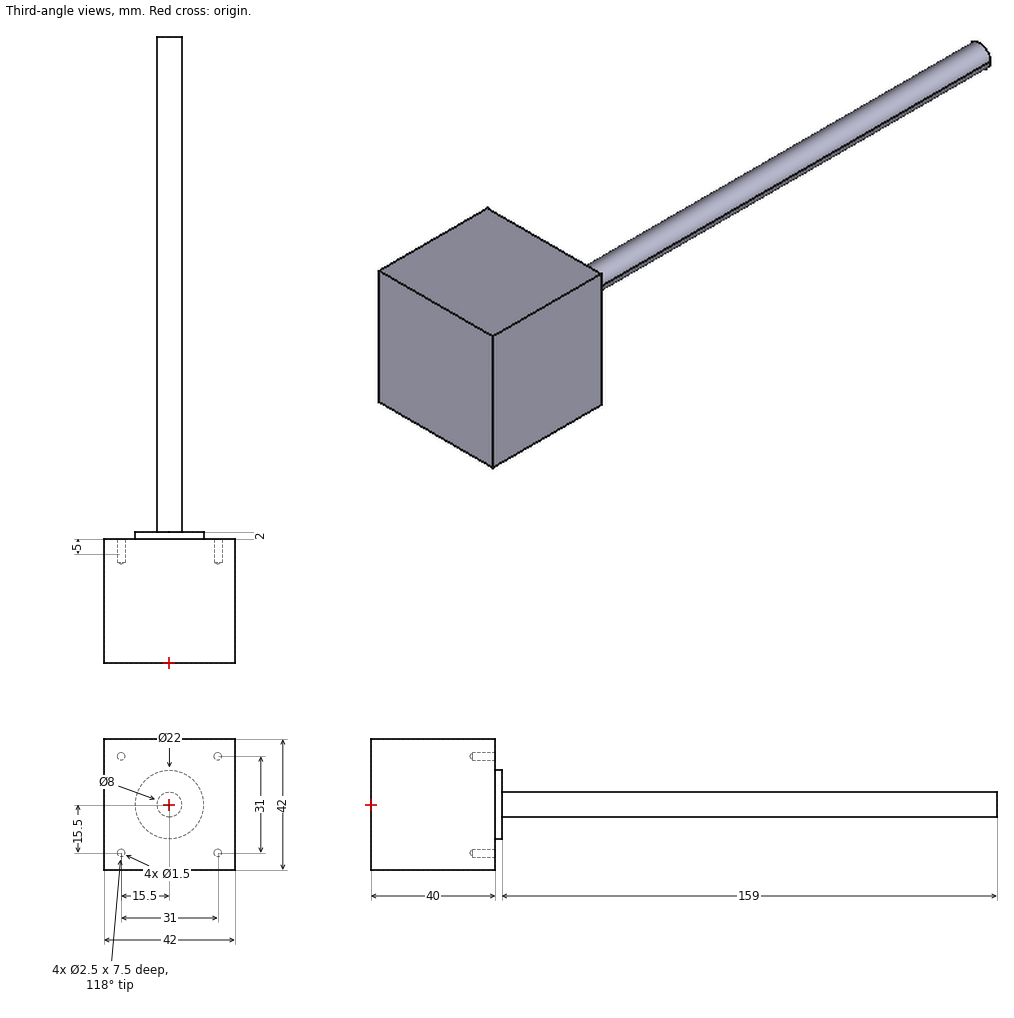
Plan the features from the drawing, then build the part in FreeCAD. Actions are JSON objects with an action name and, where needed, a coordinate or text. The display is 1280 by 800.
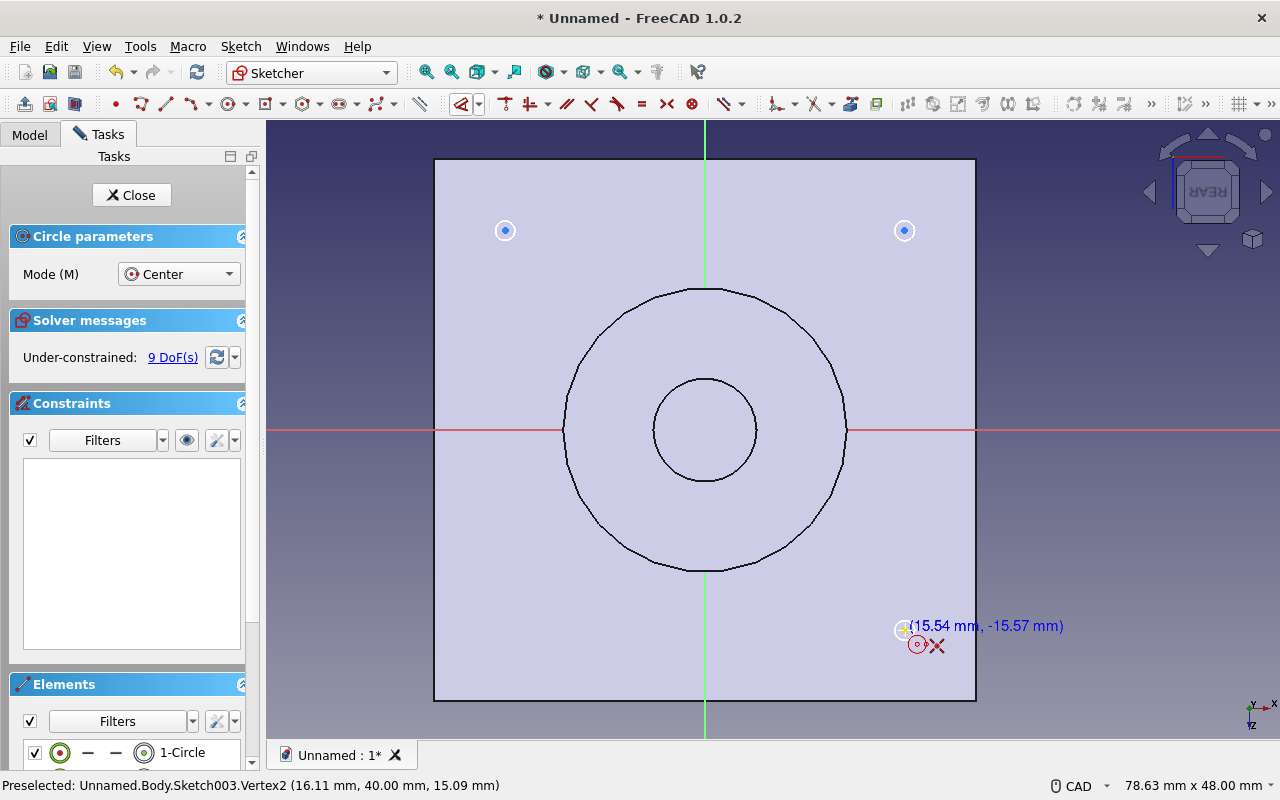
{"action": "scroll", "coordinate": [505, 630], "scroll_direction": "up", "scroll_amount": 5}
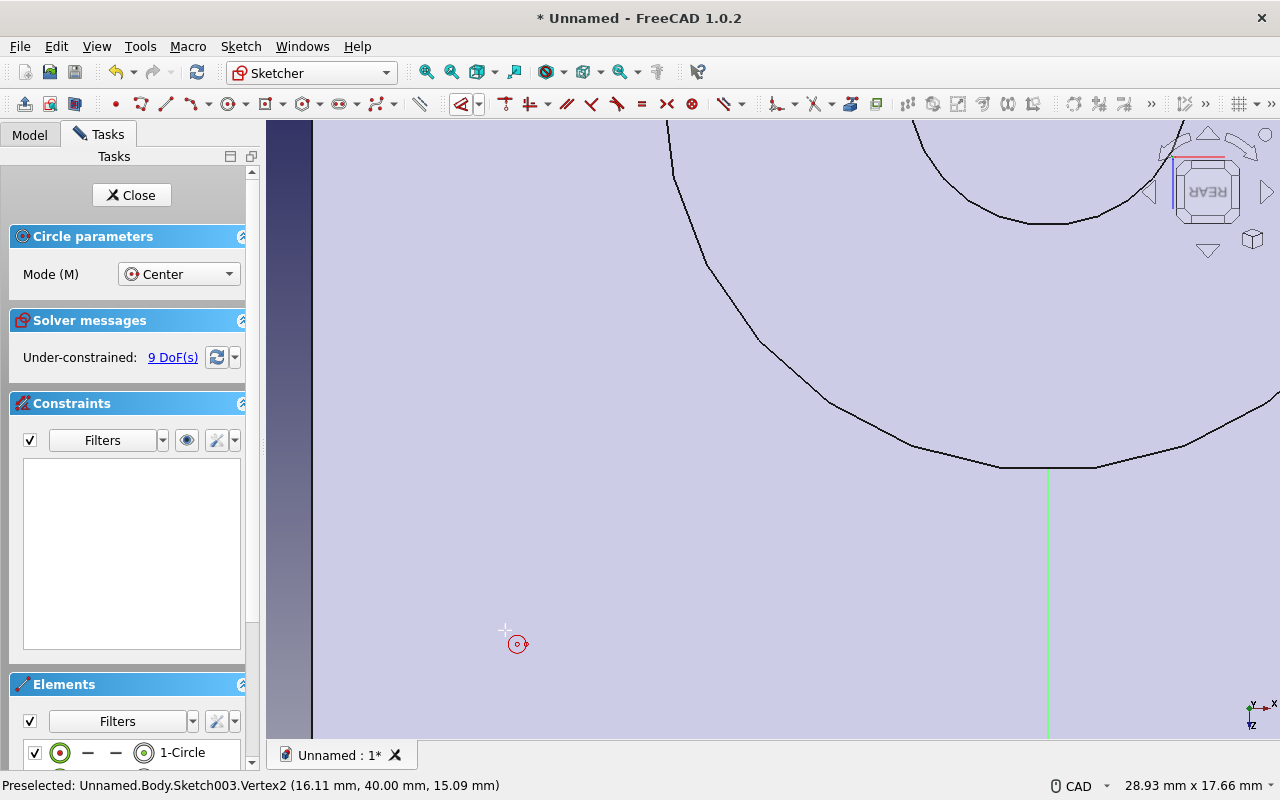
{"action": "left_click", "coordinate": [505, 629]}
{"action": "left_click", "coordinate": [523, 610]}
{"action": "key", "text": "Escape"}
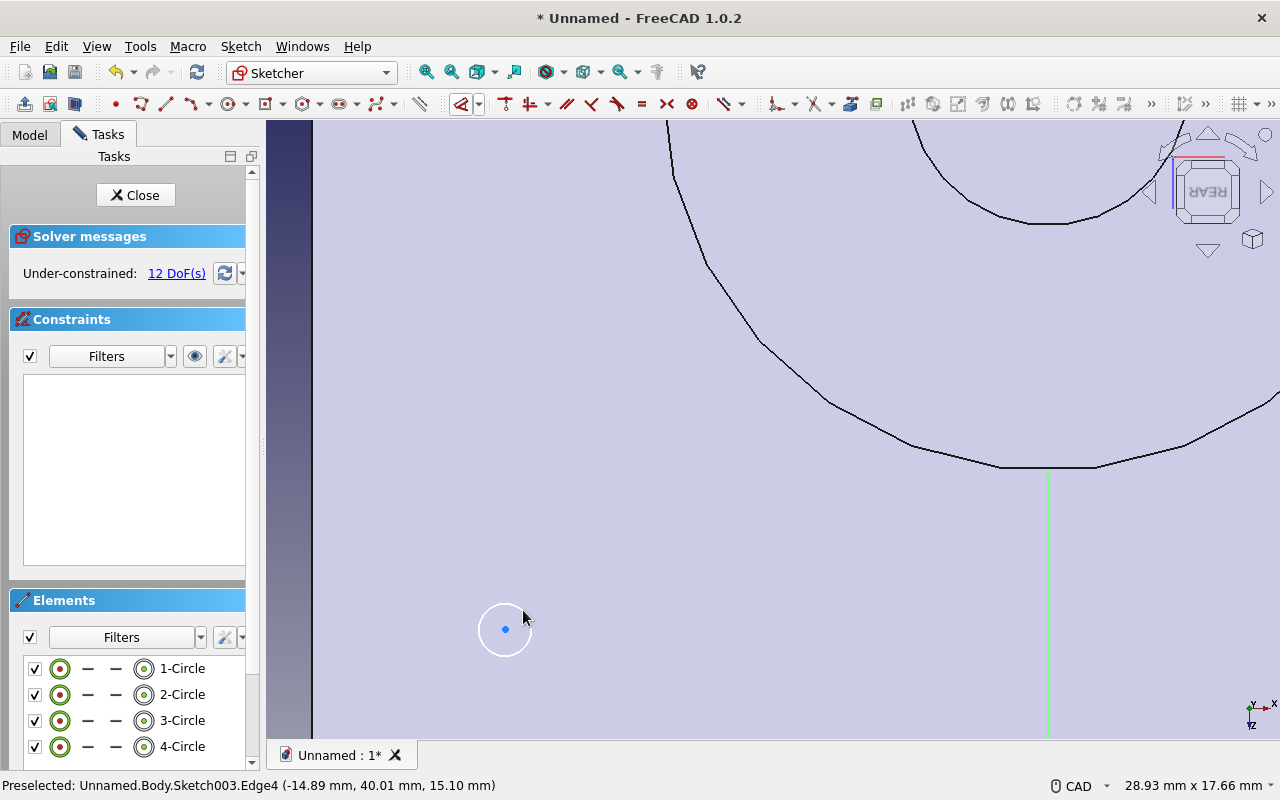
{"action": "scroll", "coordinate": [505, 630], "scroll_direction": "down", "scroll_amount": 5}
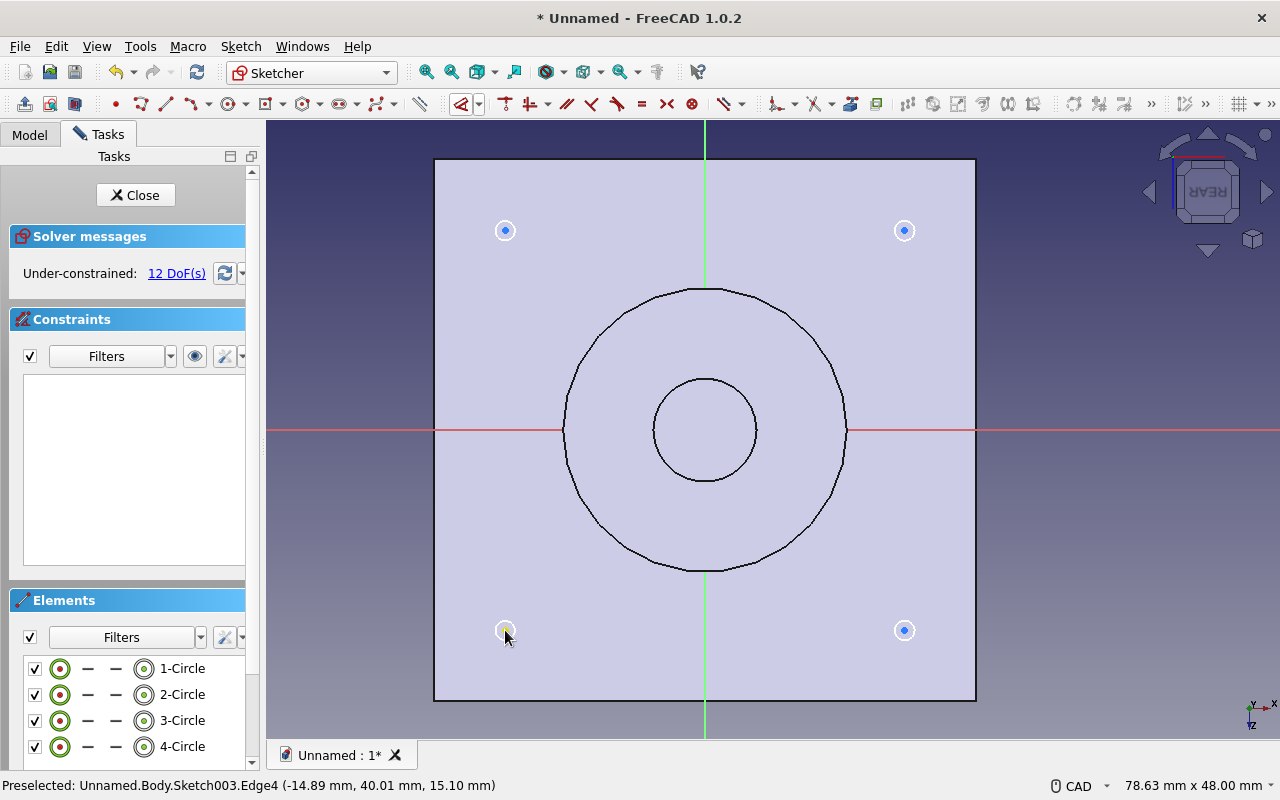
{"action": "scroll", "coordinate": [512, 224], "scroll_direction": "up", "scroll_amount": 2}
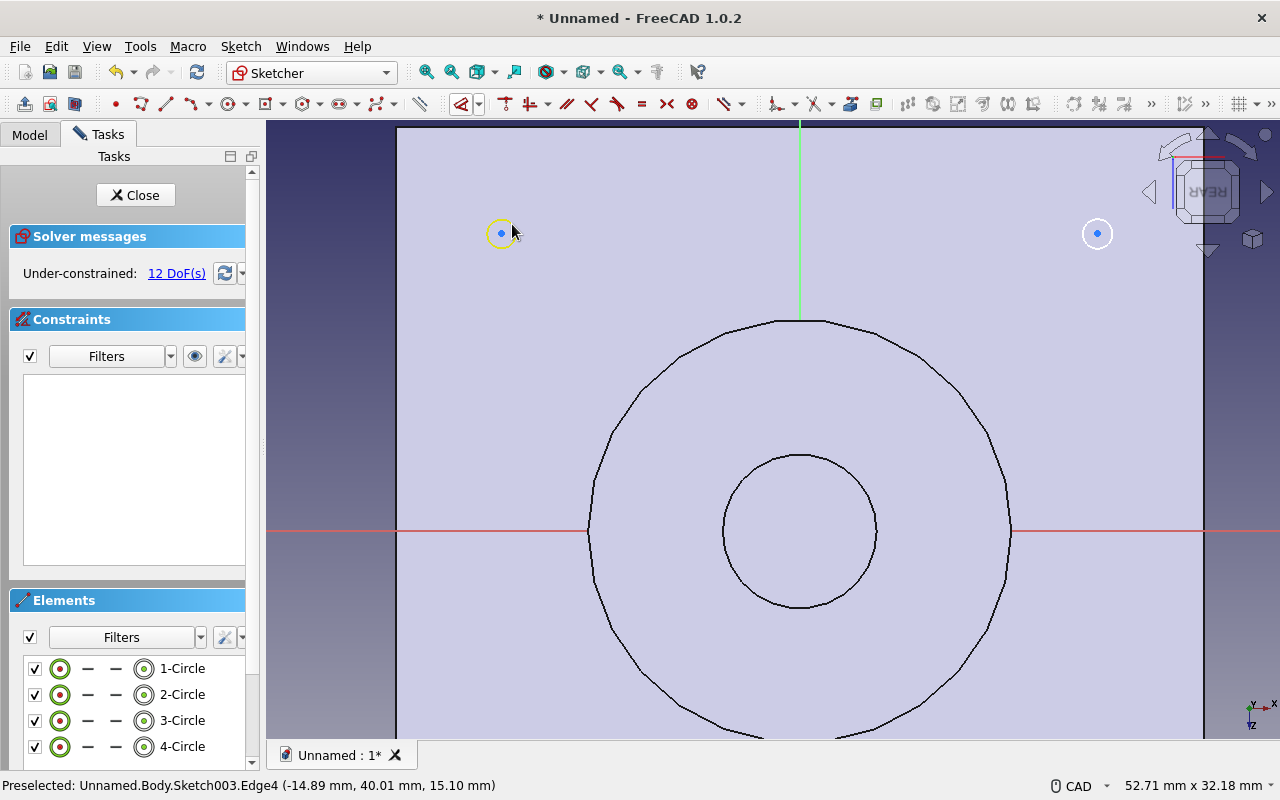
{"action": "left_click", "coordinate": [512, 224]}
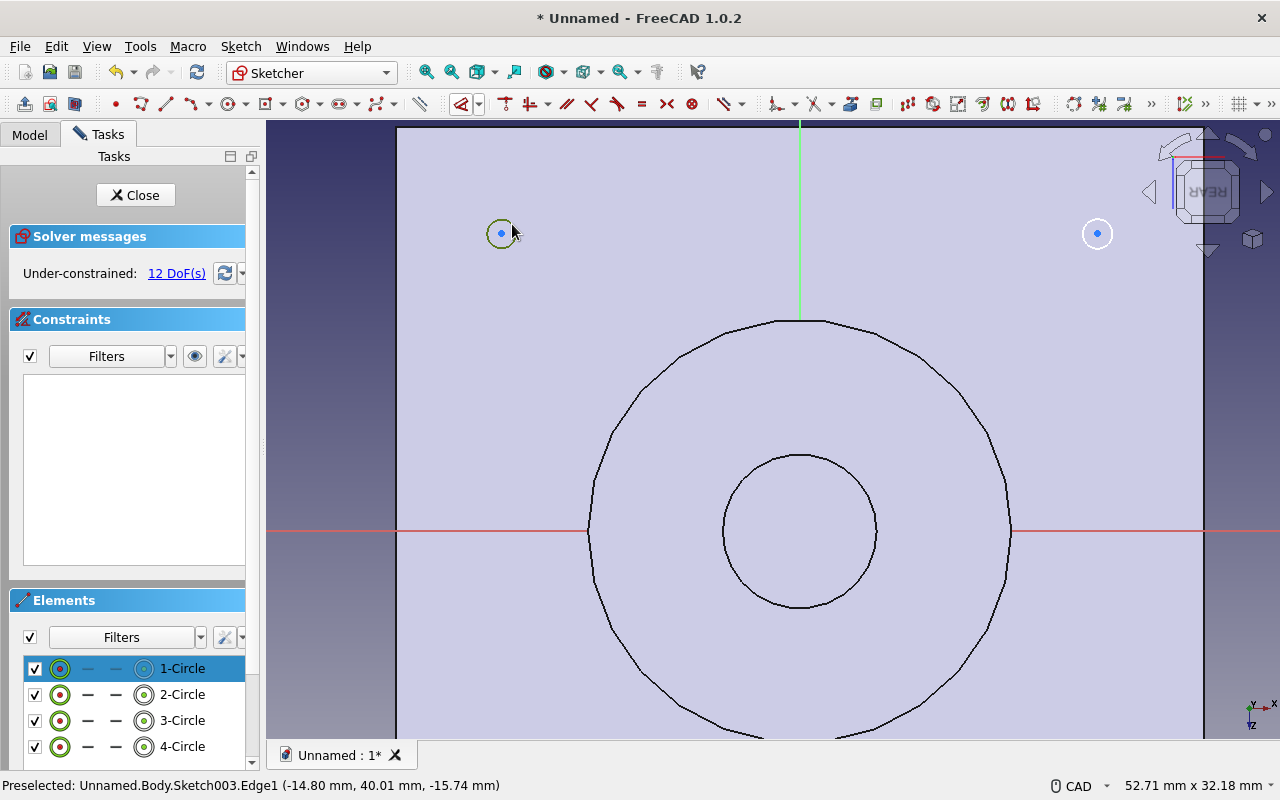
{"action": "left_click", "coordinate": [1108, 224]}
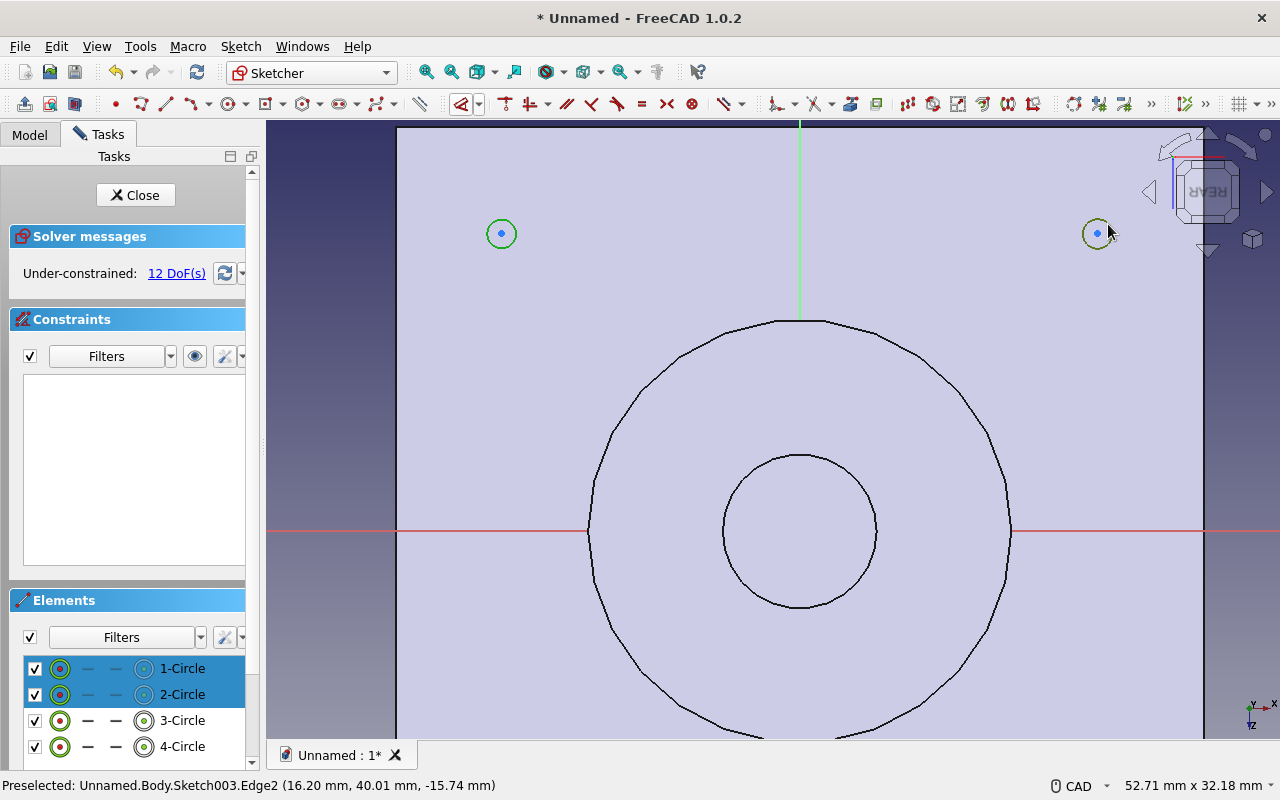
{"action": "scroll", "coordinate": [511, 222], "scroll_direction": "down", "scroll_amount": 2}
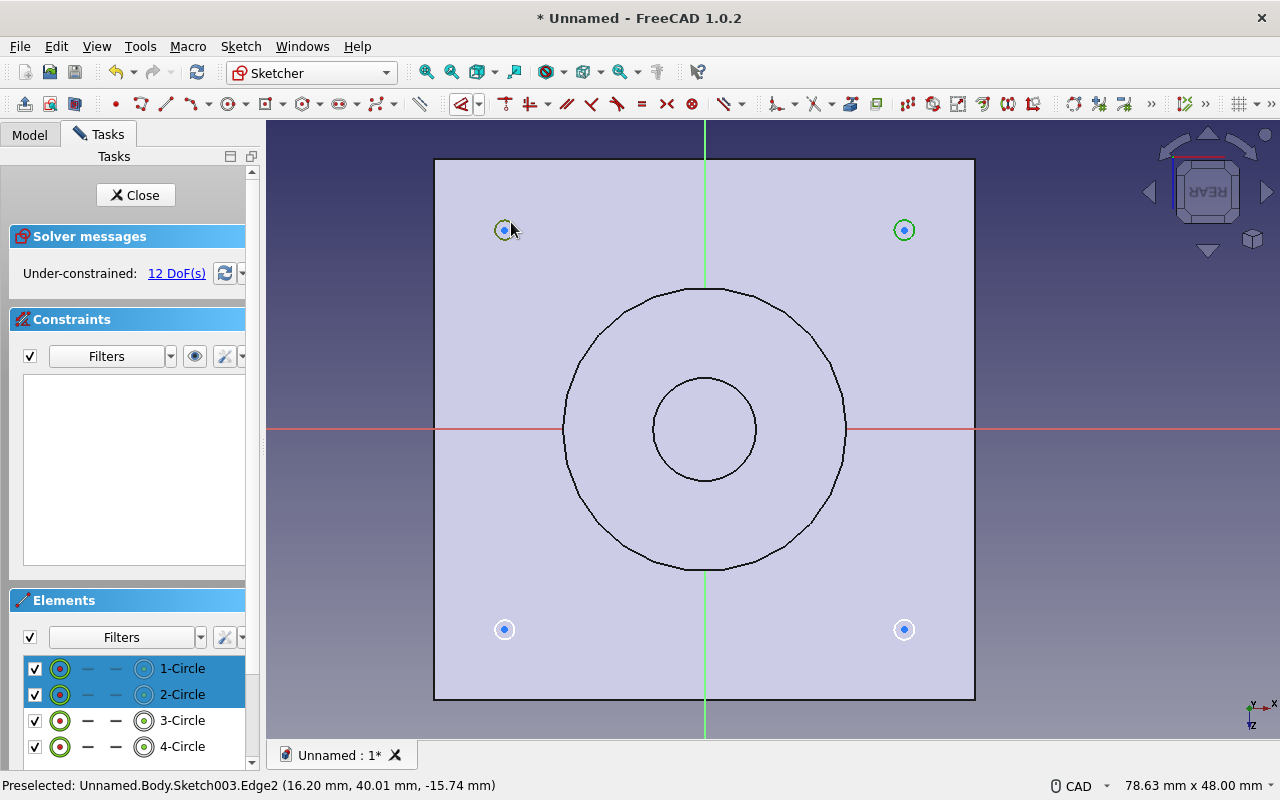
{"action": "scroll", "coordinate": [911, 623], "scroll_direction": "up", "scroll_amount": 2}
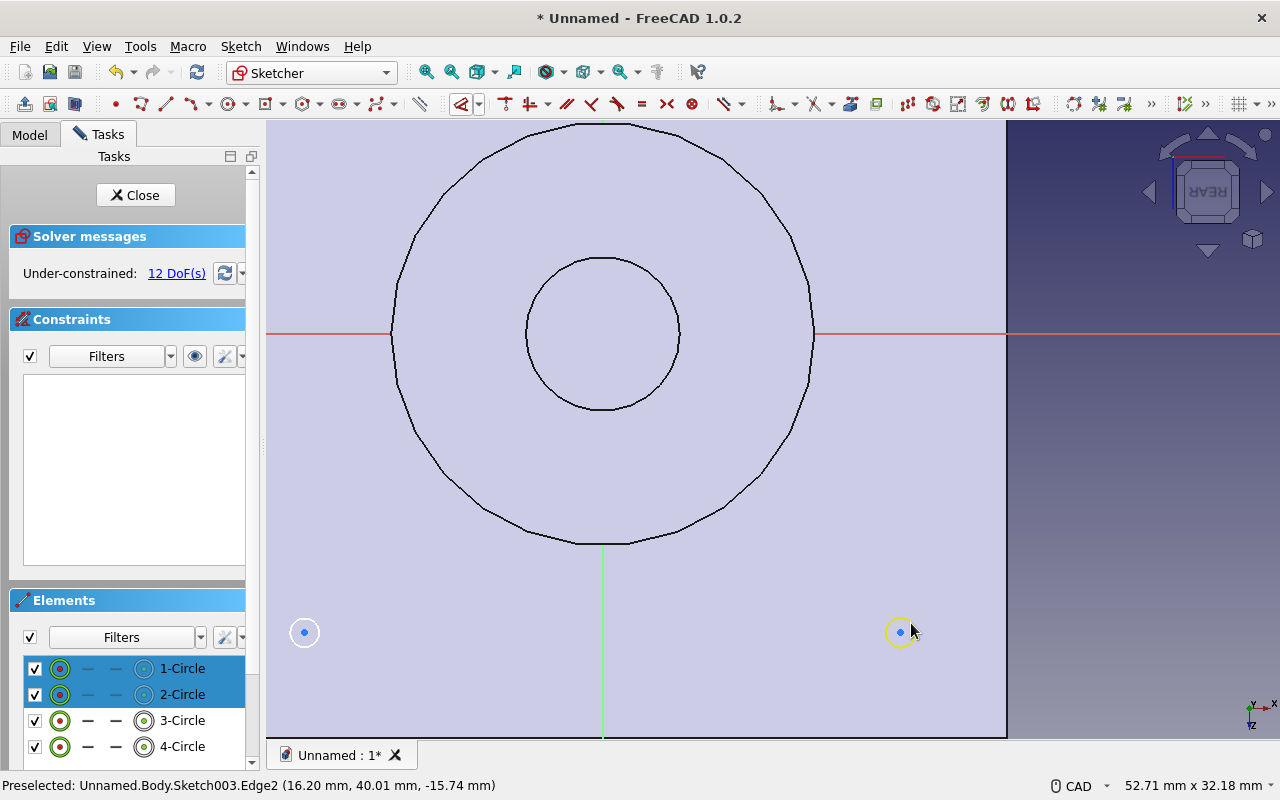
{"action": "left_click", "coordinate": [911, 622]}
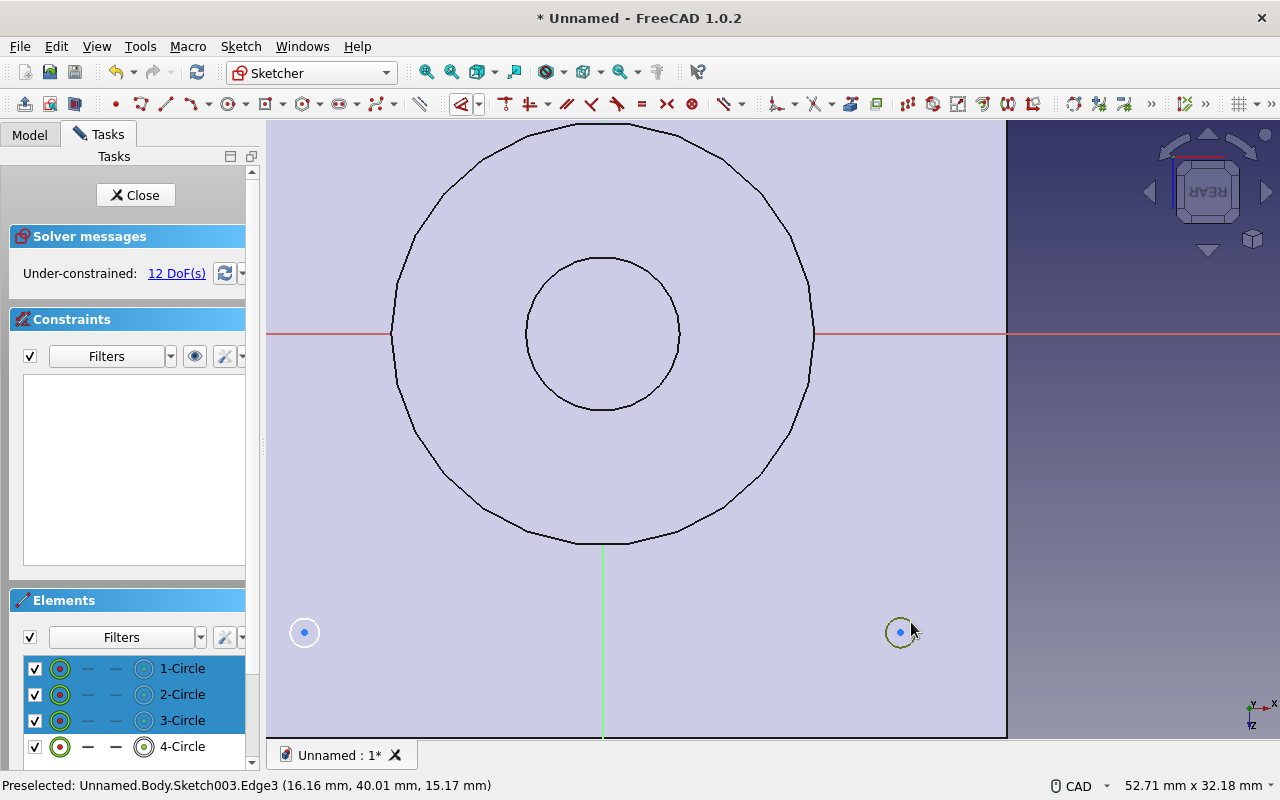
{"action": "left_click", "coordinate": [315, 623]}